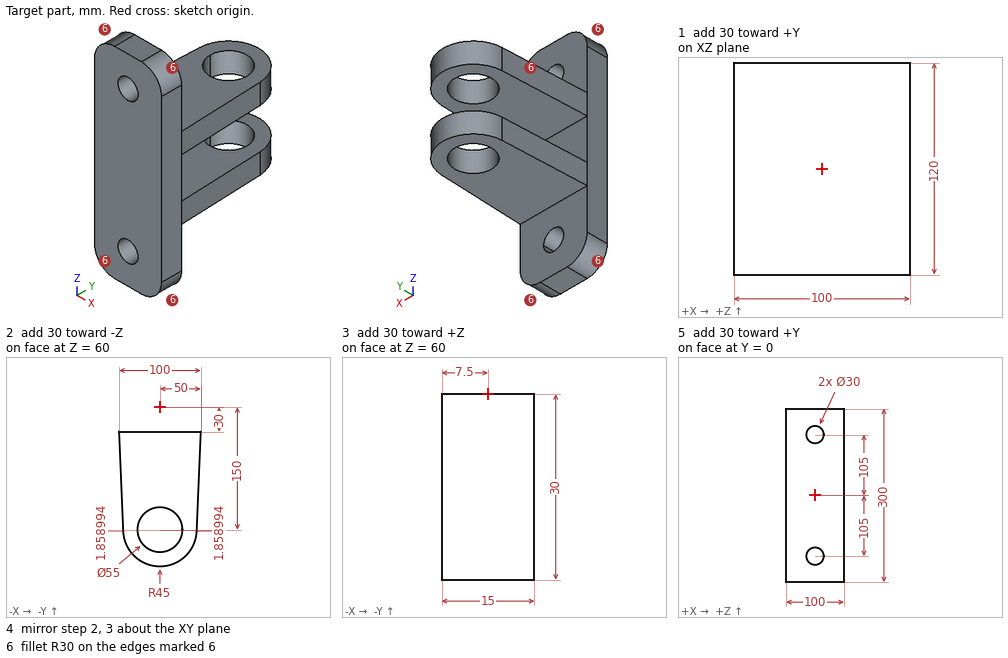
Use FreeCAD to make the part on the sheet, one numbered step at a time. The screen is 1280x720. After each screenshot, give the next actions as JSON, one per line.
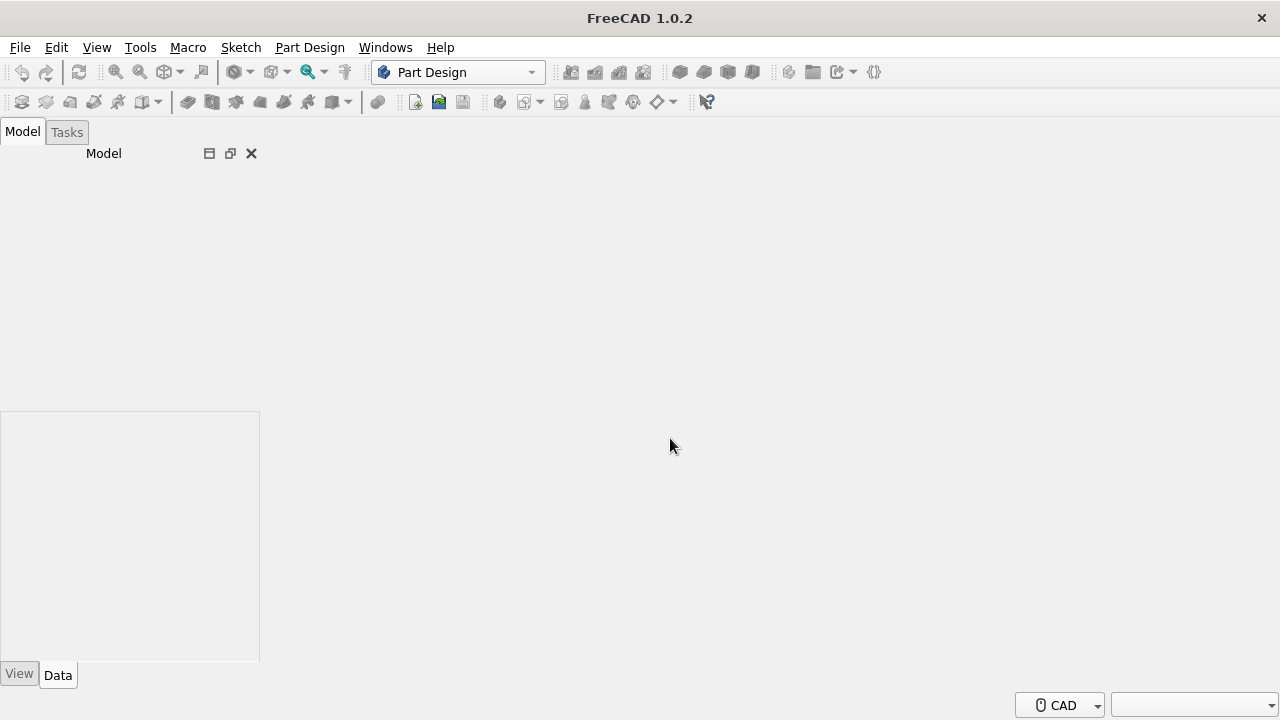
{"action": "left_click", "coordinate": [416, 102]}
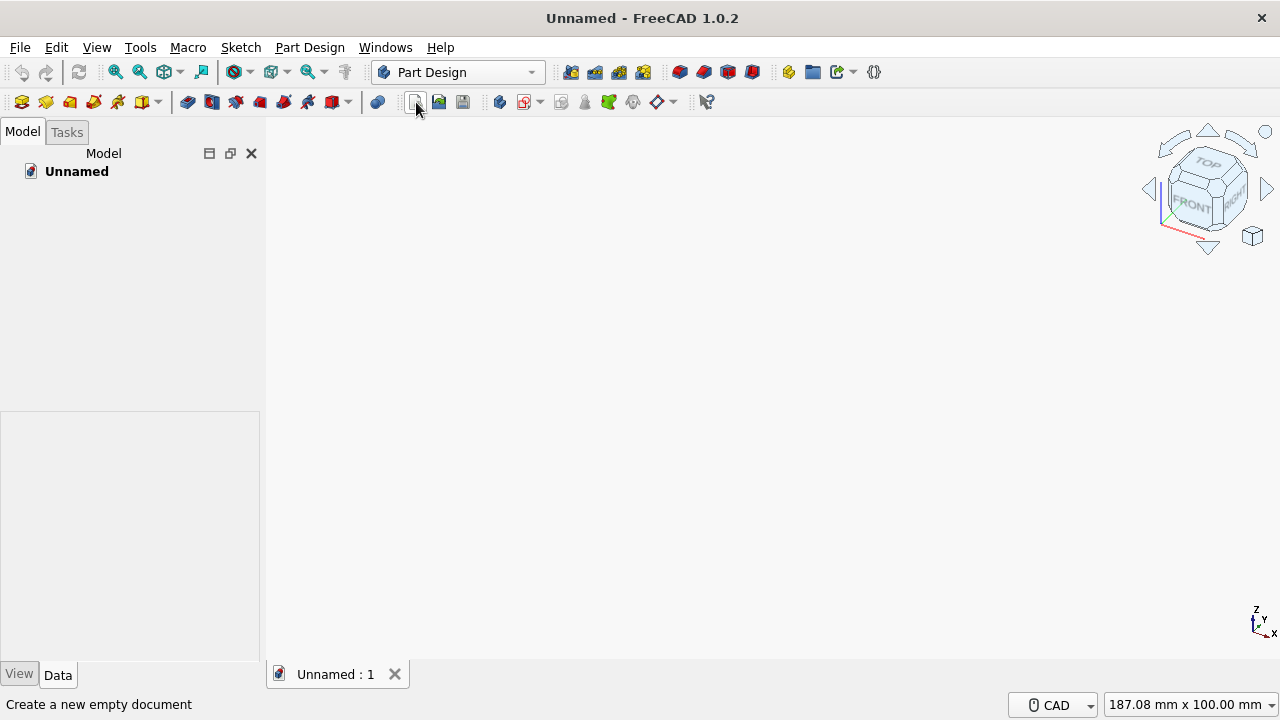
{"action": "left_click", "coordinate": [524, 102]}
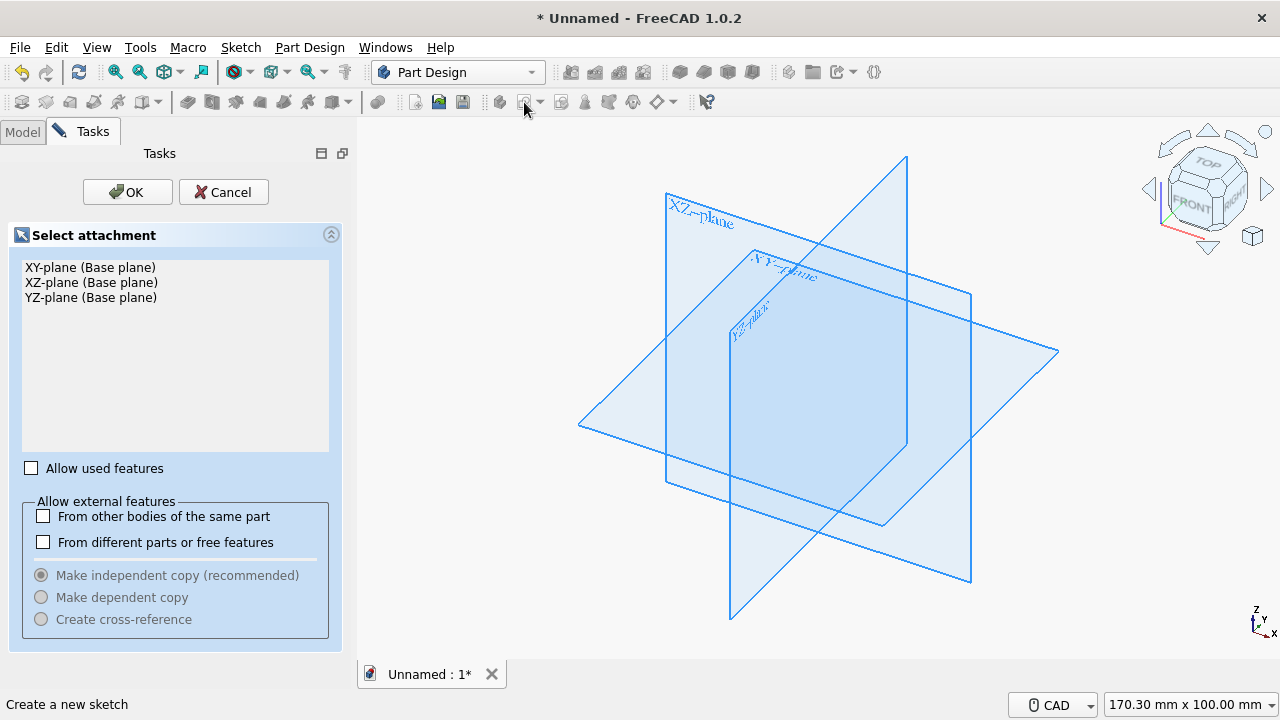
{"action": "left_click", "coordinate": [82, 282]}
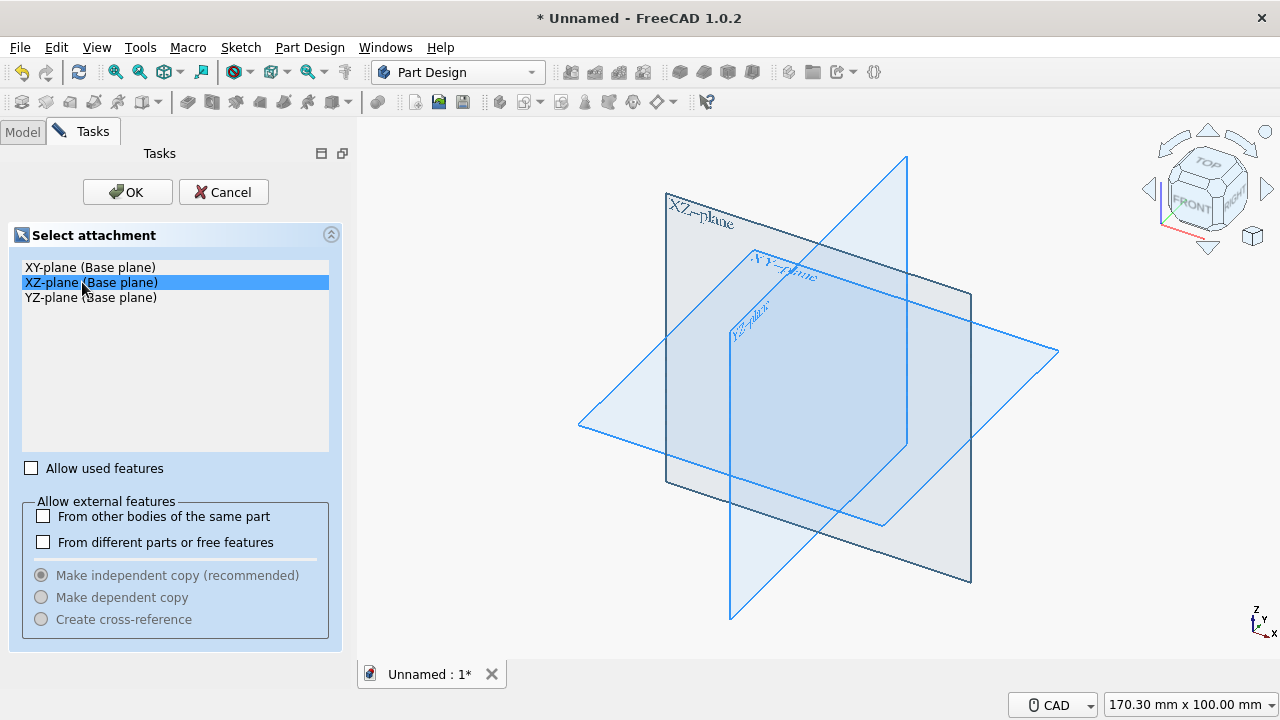
{"action": "left_click", "coordinate": [128, 192]}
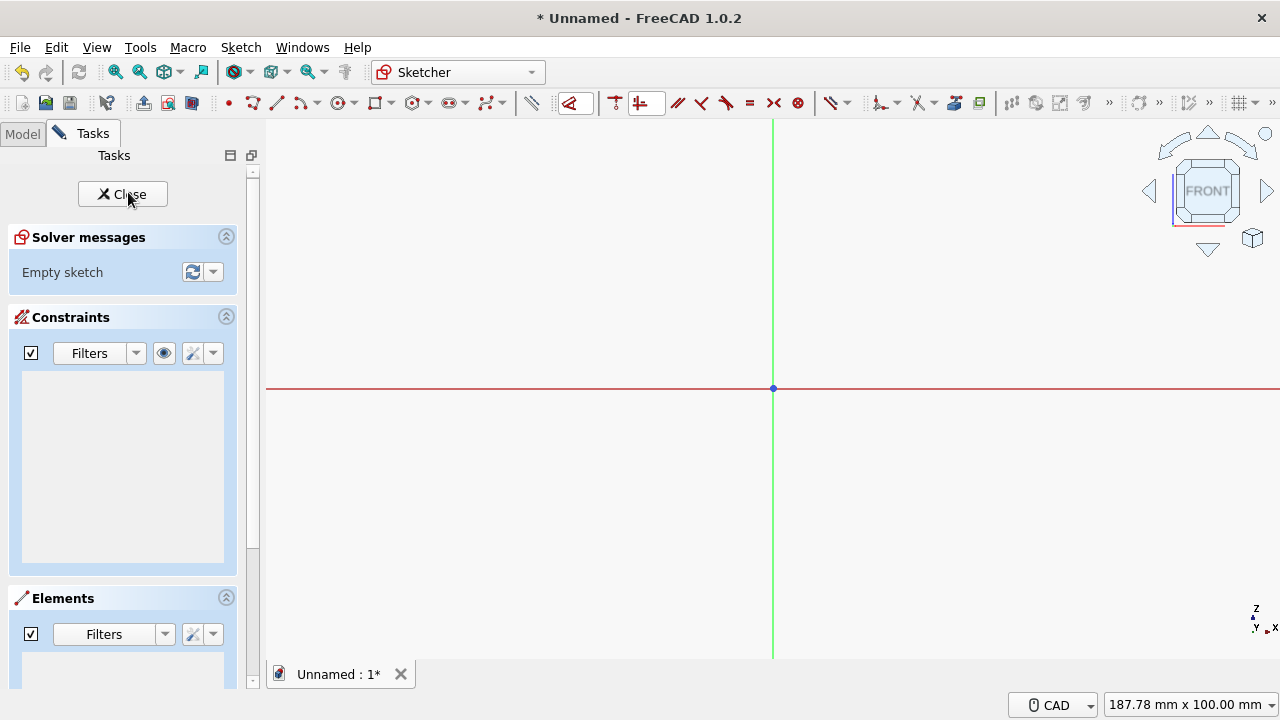
{"action": "scroll", "coordinate": [621, 389], "scroll_direction": "down", "scroll_amount": 3}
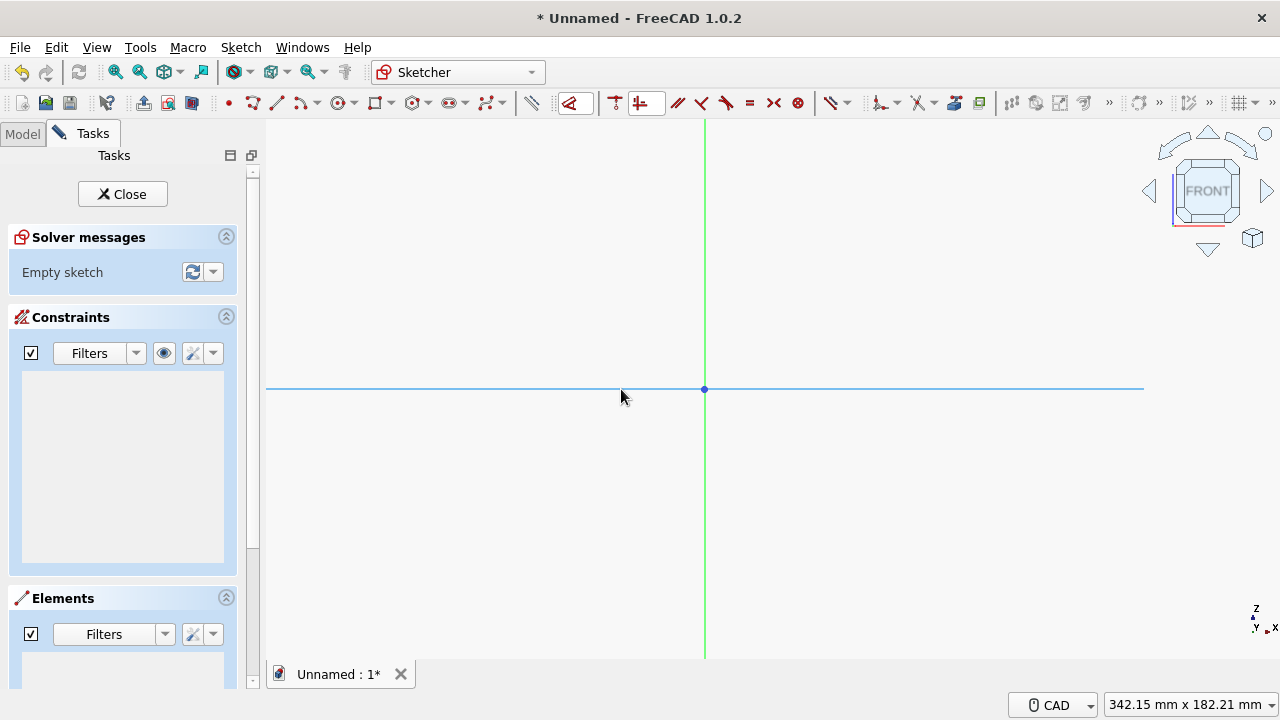
{"action": "key", "text": "g v"}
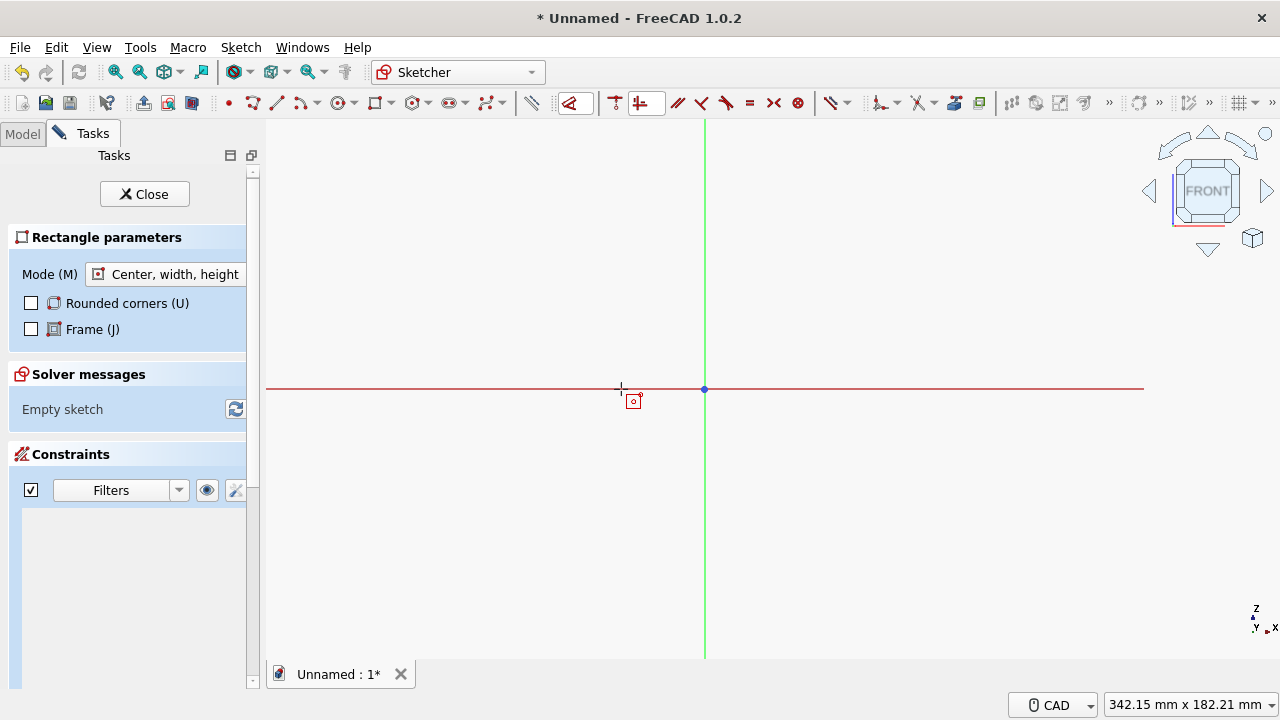
{"action": "left_click", "coordinate": [705, 389]}
{"action": "mouse_move", "coordinate": [853, 211]}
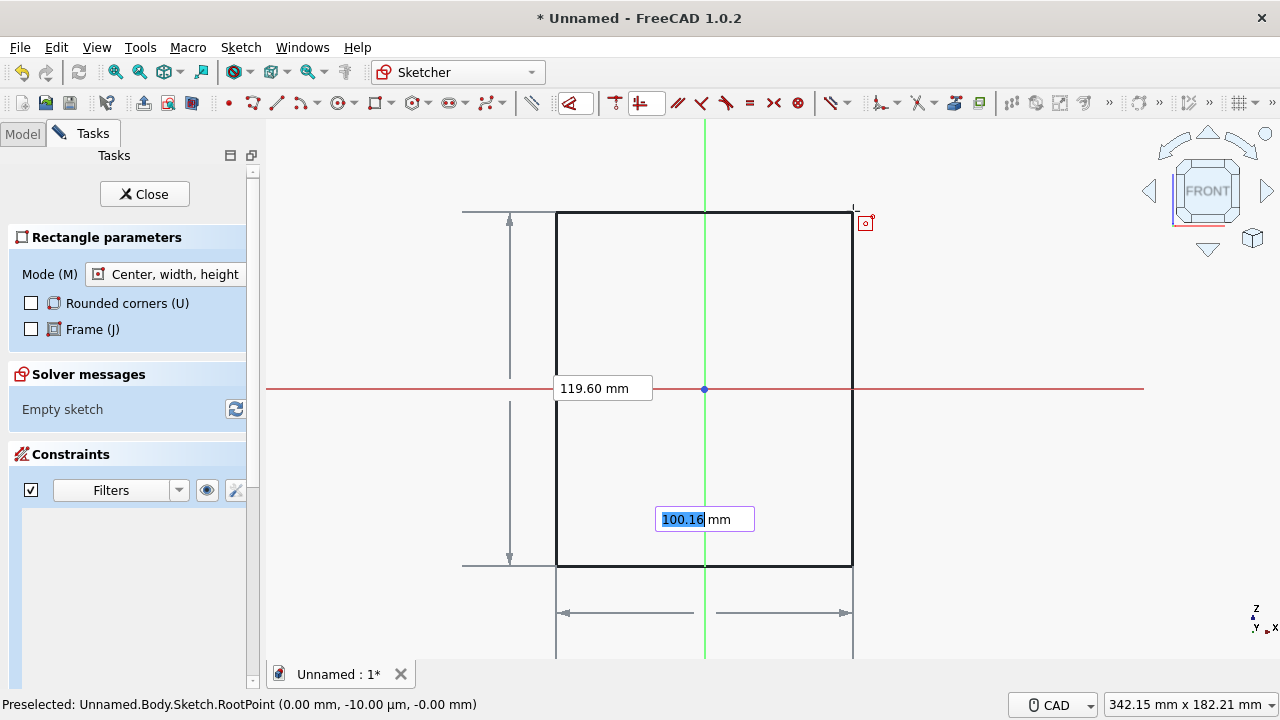
{"action": "type", "text": "100"}
{"action": "key", "text": "Tab"}
{"action": "type", "text": "120"}
{"action": "key", "text": "Return"}
{"action": "key", "text": "Escape"}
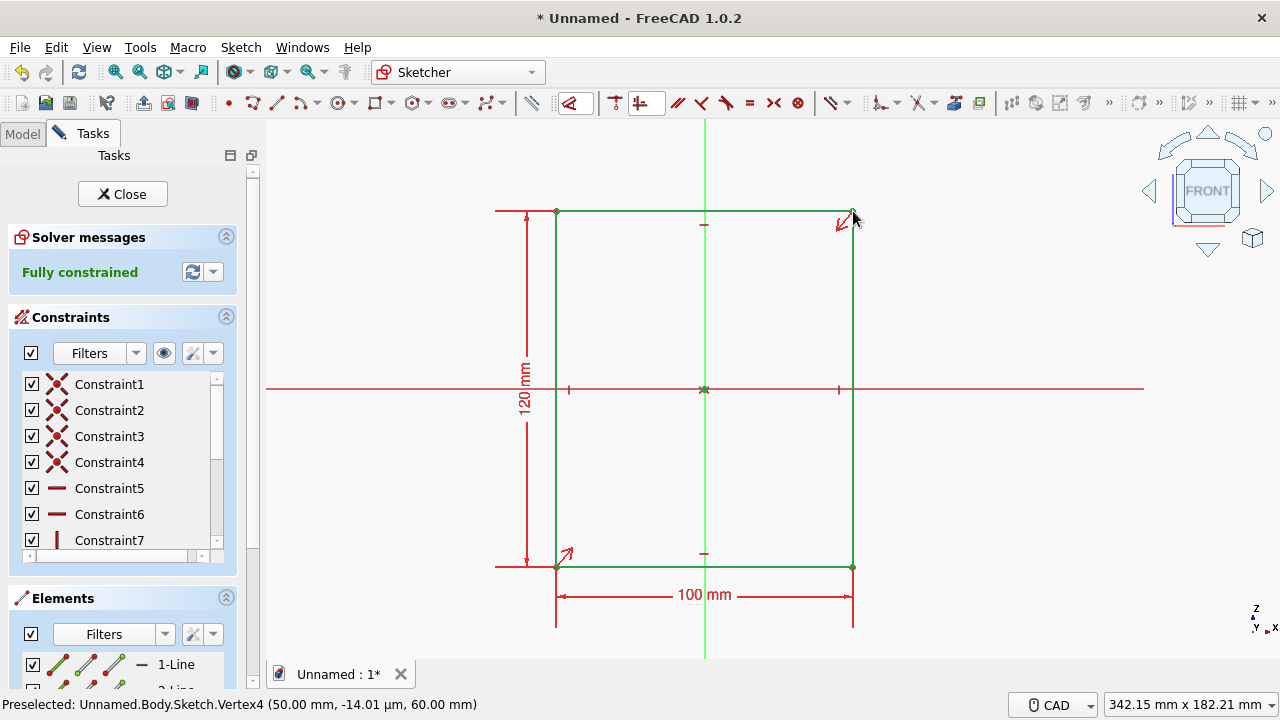
{"action": "left_click", "coordinate": [123, 194]}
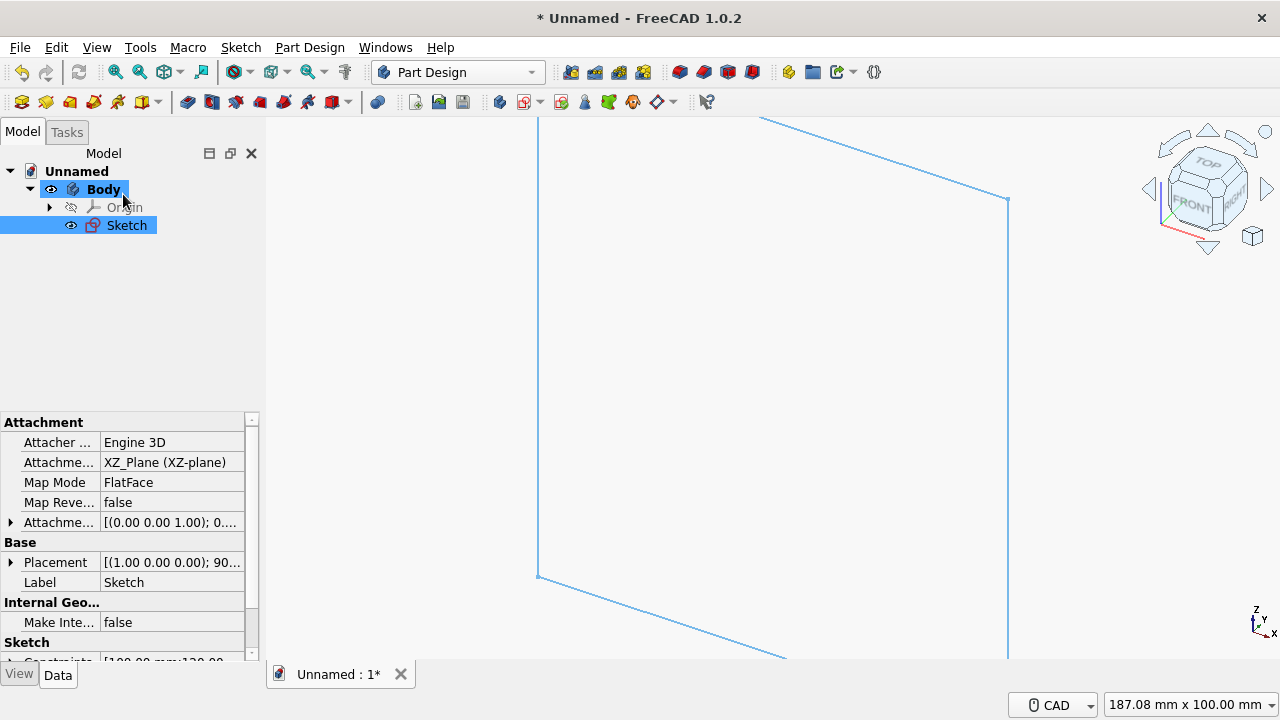
{"action": "left_click", "coordinate": [22, 102]}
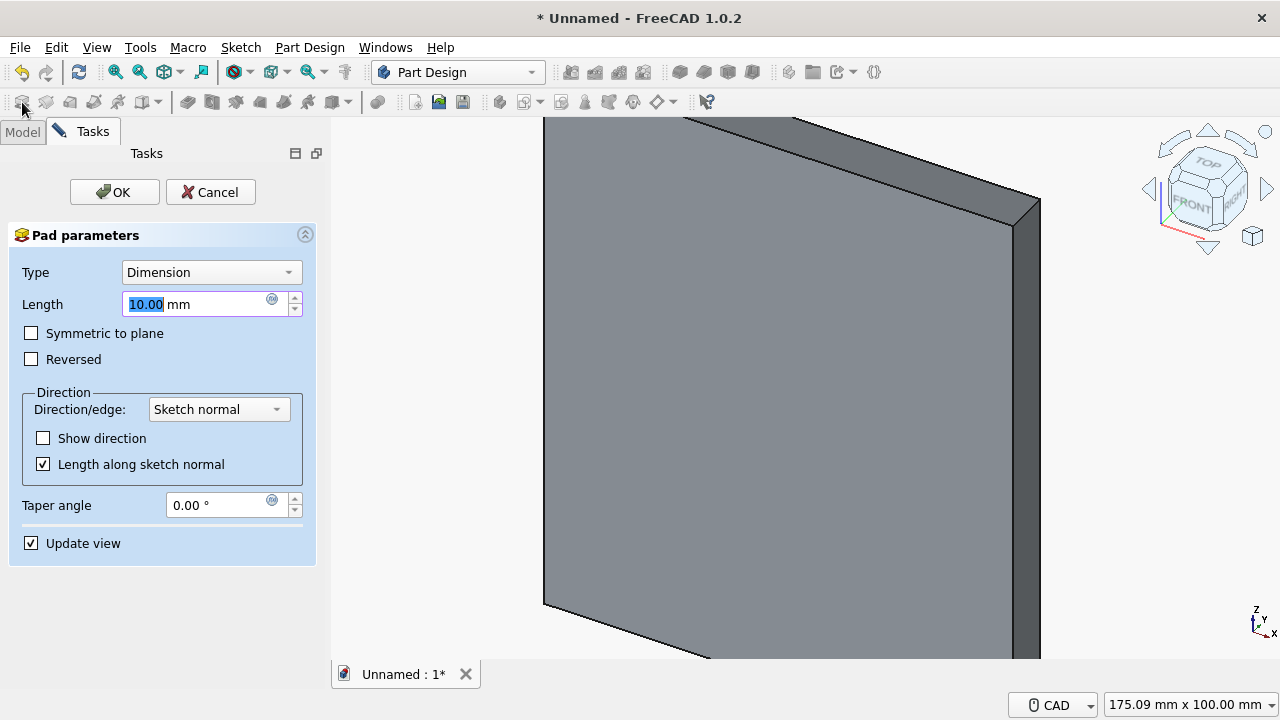
{"action": "type", "text": "30"}
{"action": "key", "text": "Tab"}